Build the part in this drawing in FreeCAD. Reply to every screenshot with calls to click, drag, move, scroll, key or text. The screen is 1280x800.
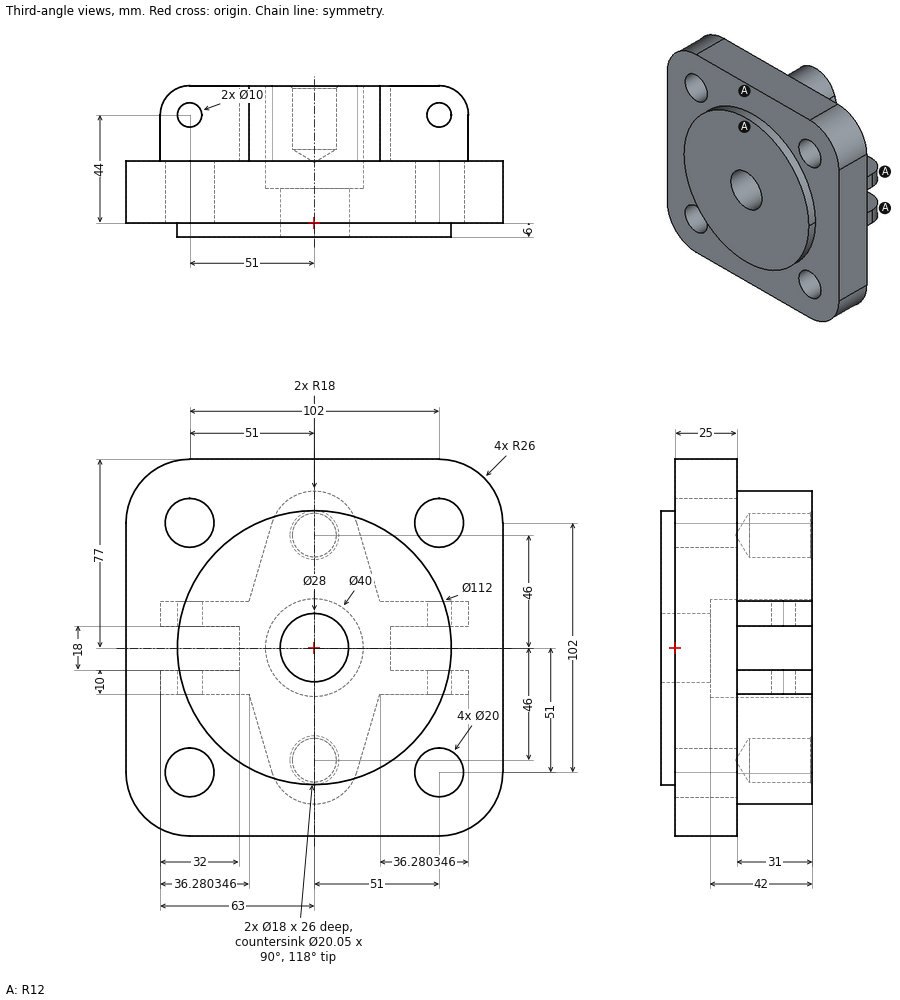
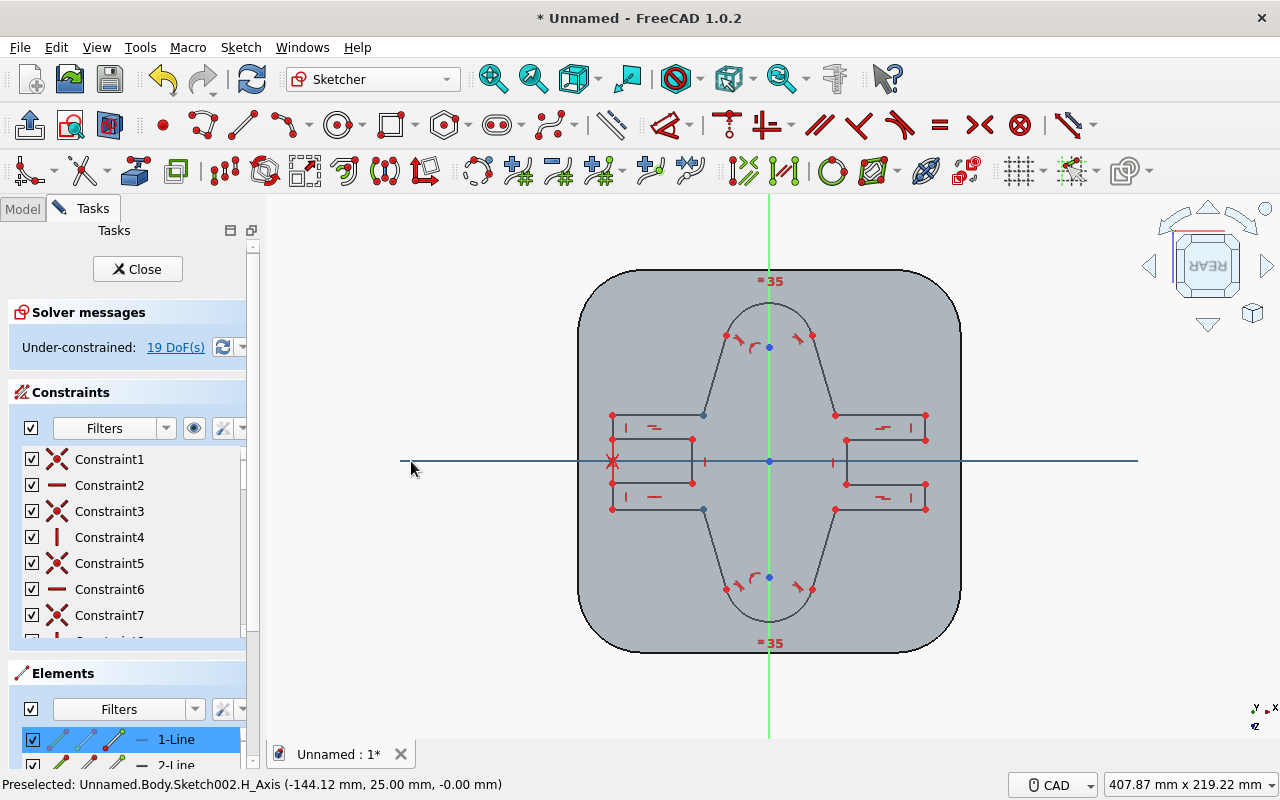
key(s)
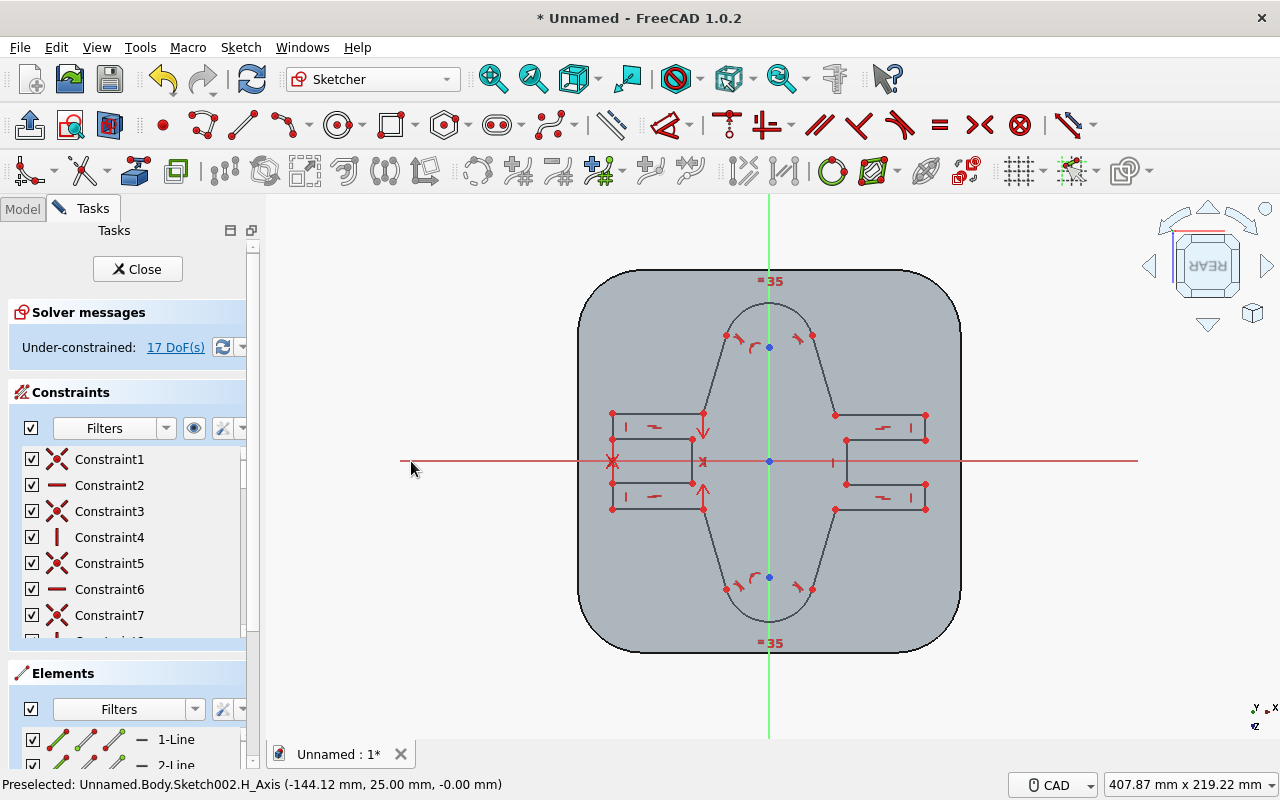
click(703, 509)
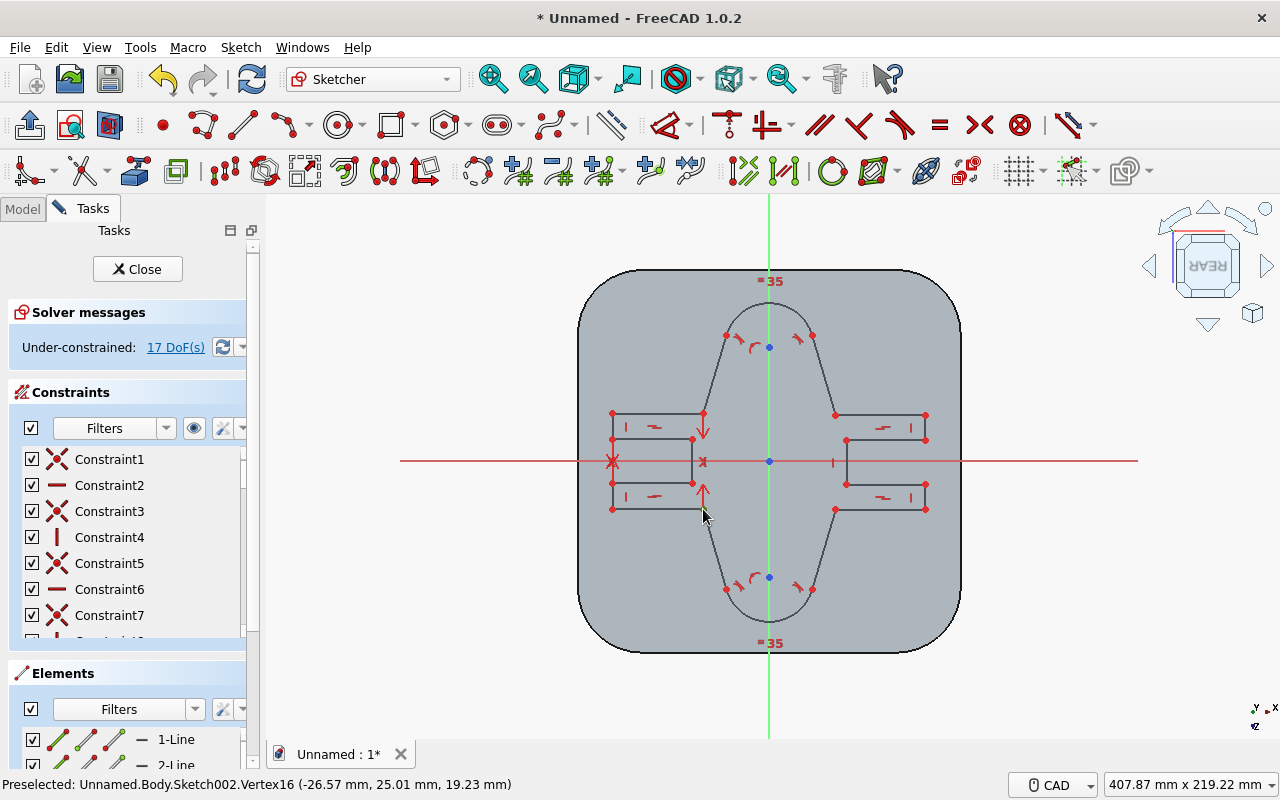
click(836, 510)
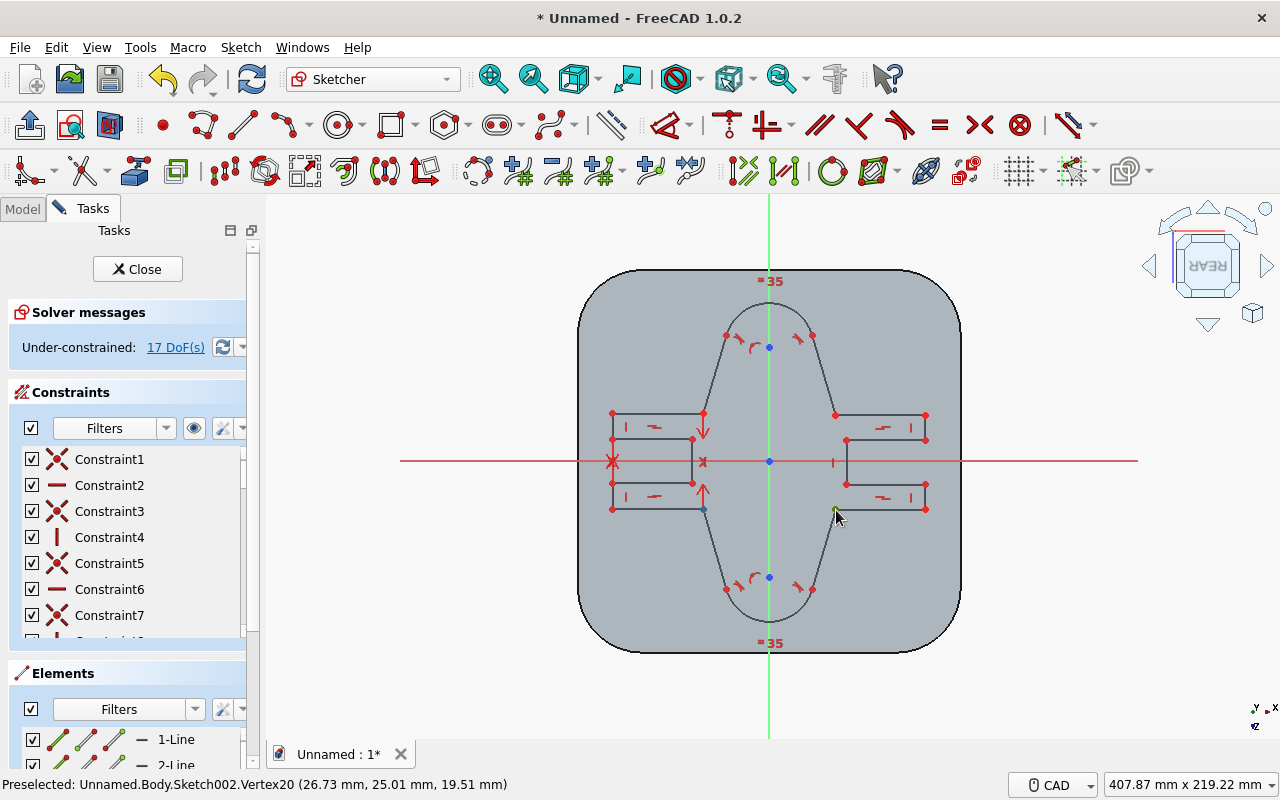
click(769, 676)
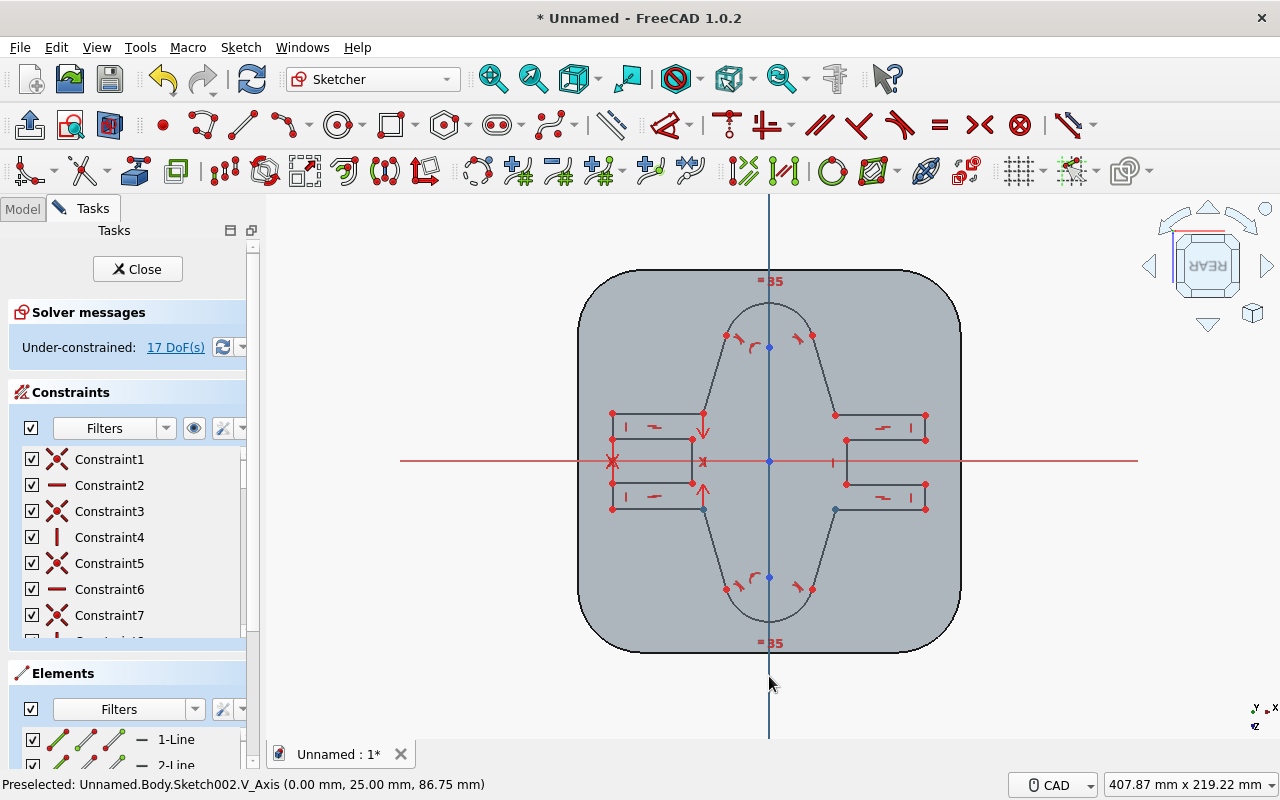
key(s)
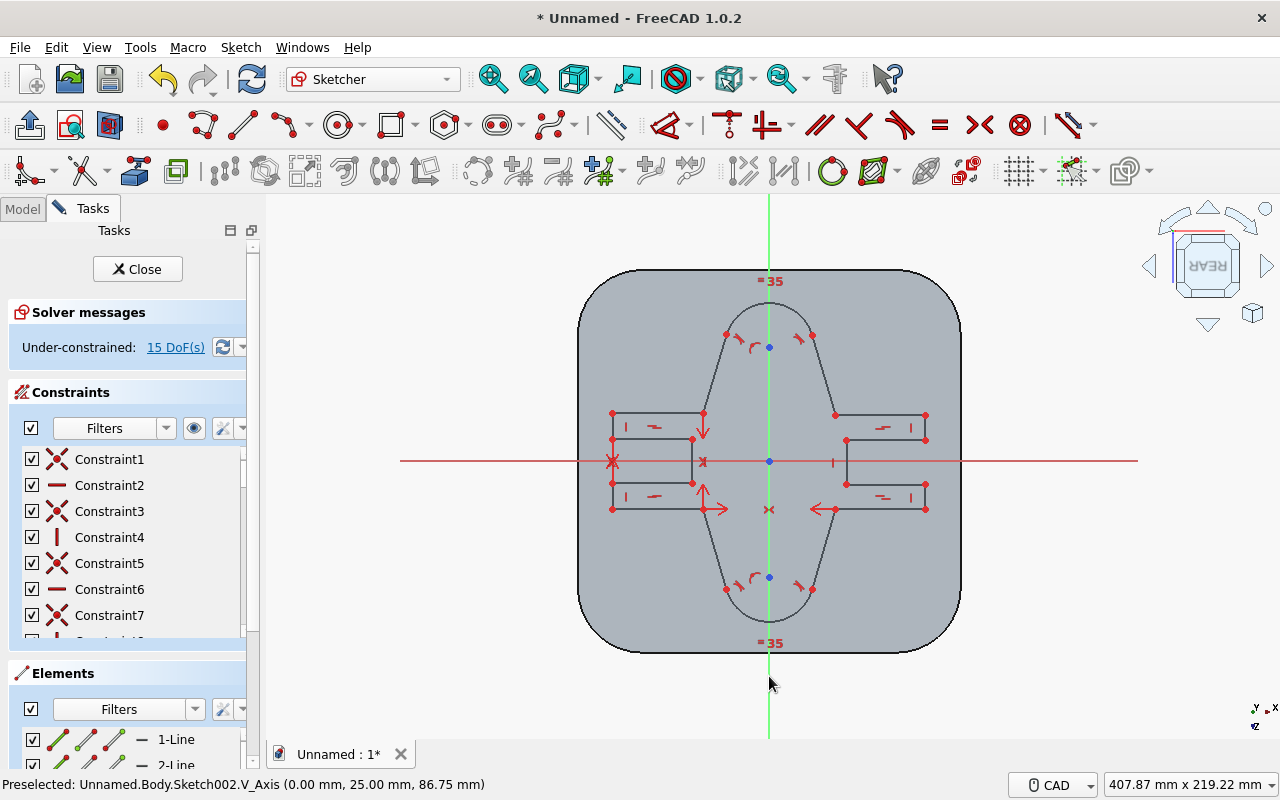
click(613, 483)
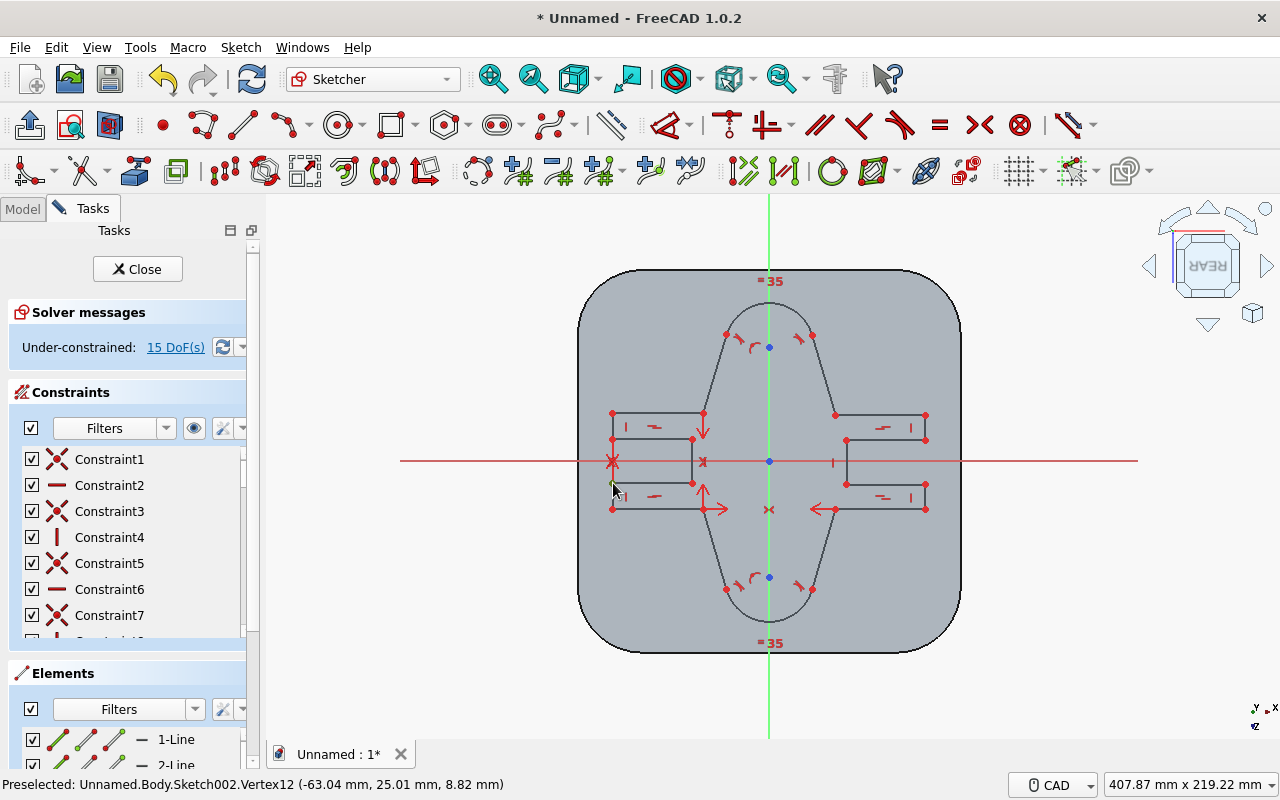
click(925, 485)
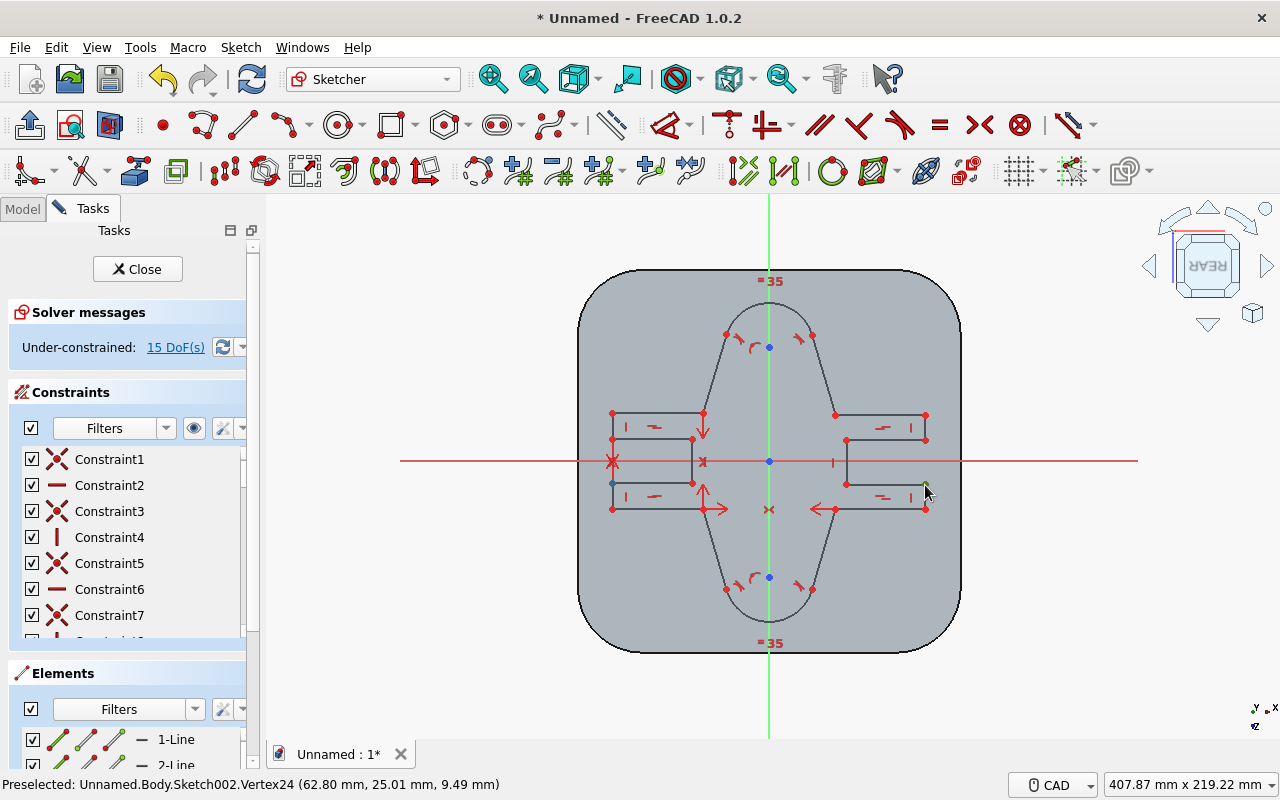
click(769, 676)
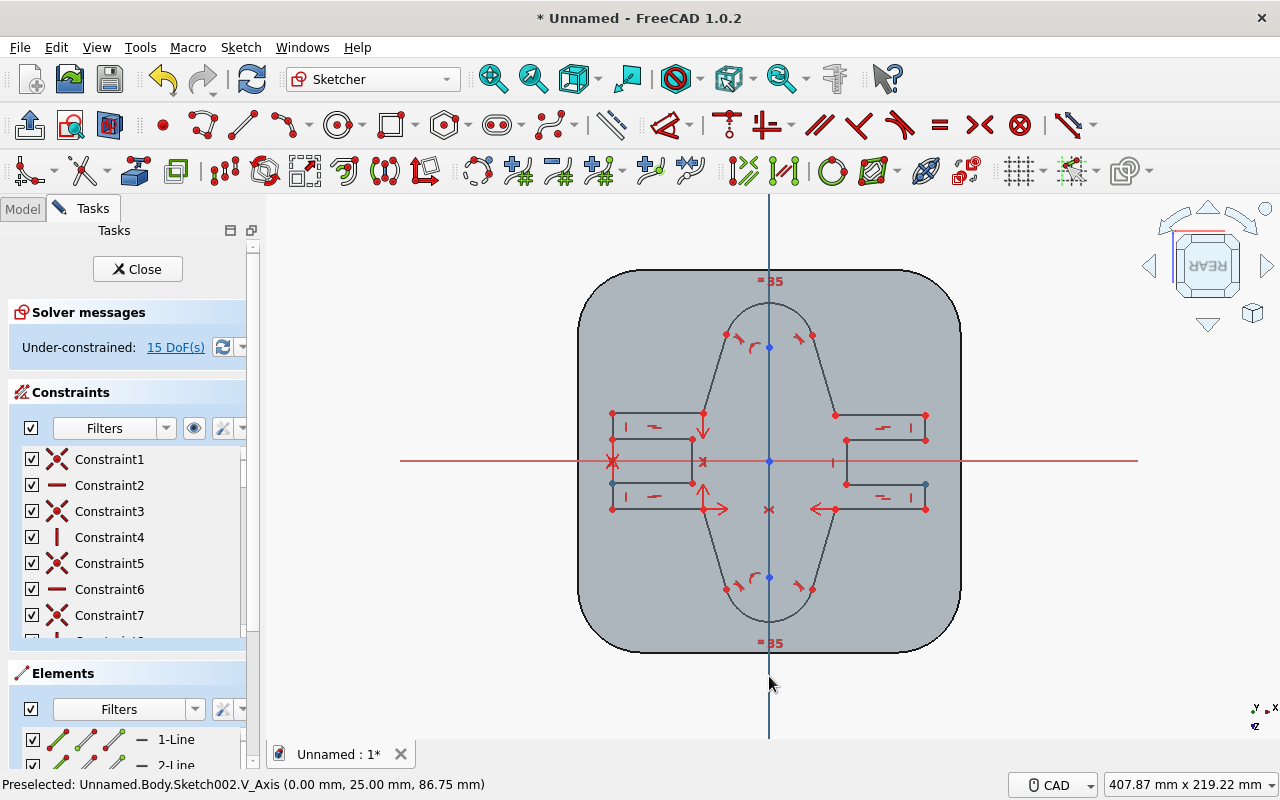
key(s)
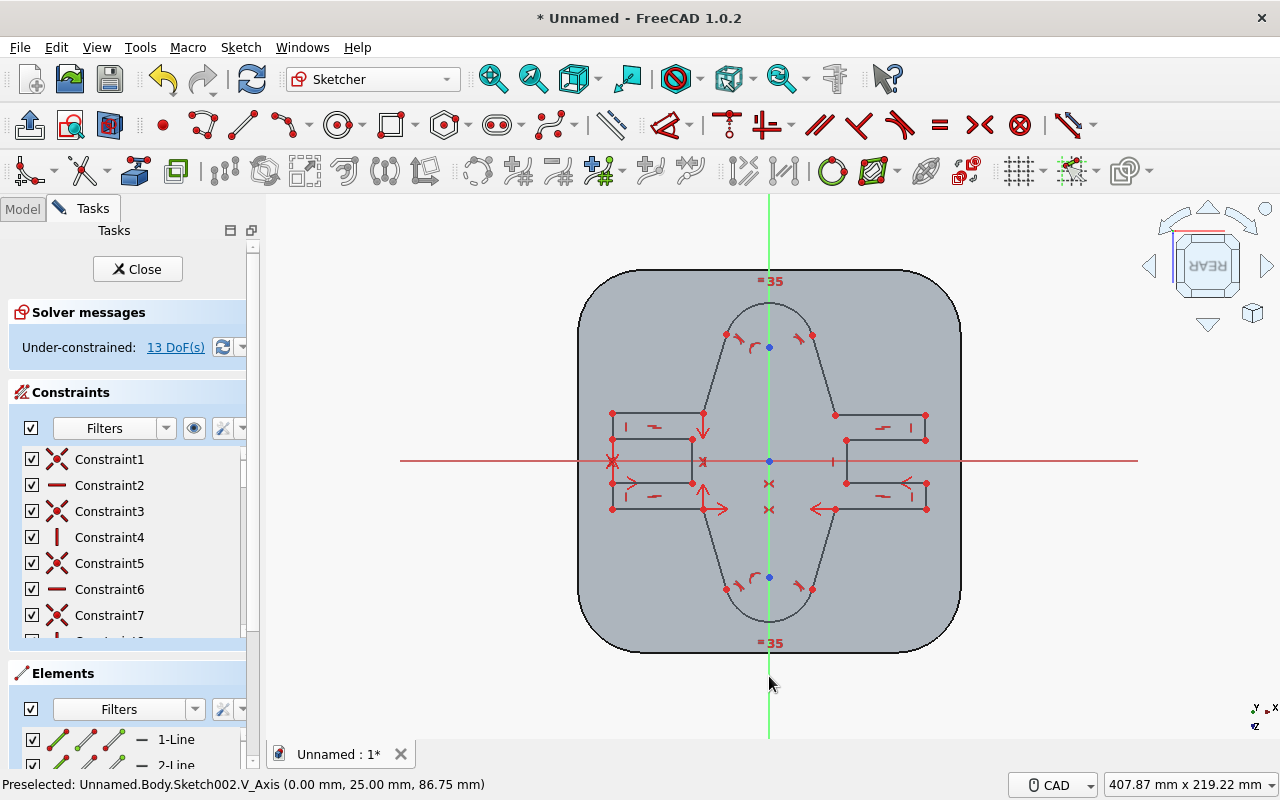
click(692, 439)